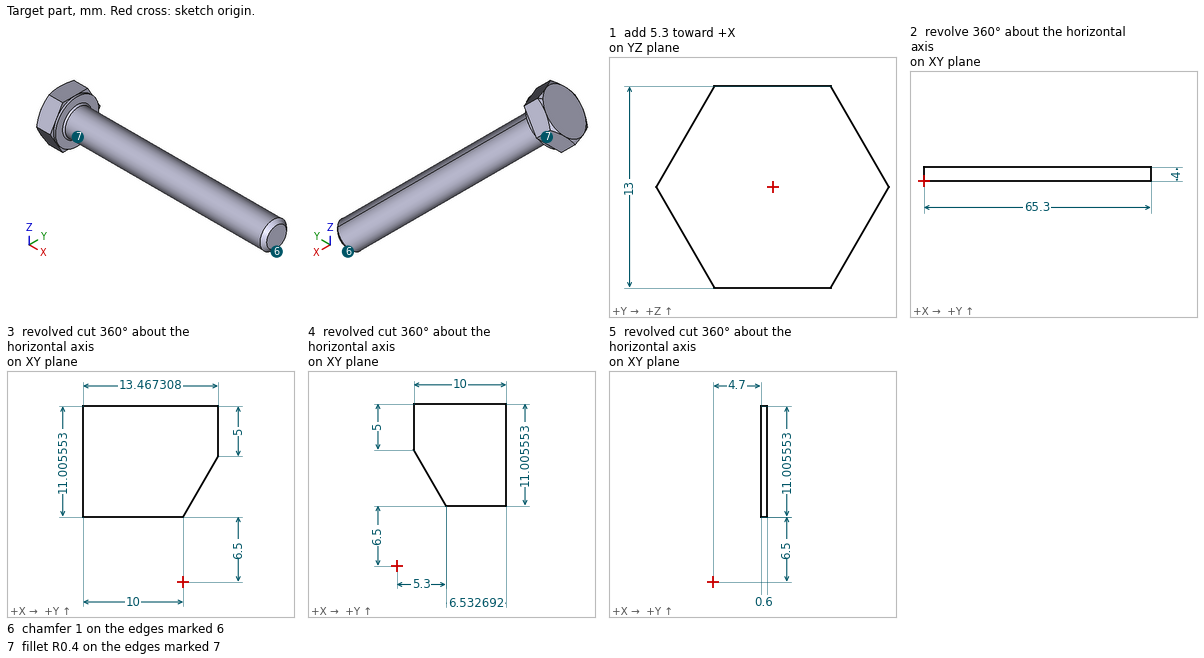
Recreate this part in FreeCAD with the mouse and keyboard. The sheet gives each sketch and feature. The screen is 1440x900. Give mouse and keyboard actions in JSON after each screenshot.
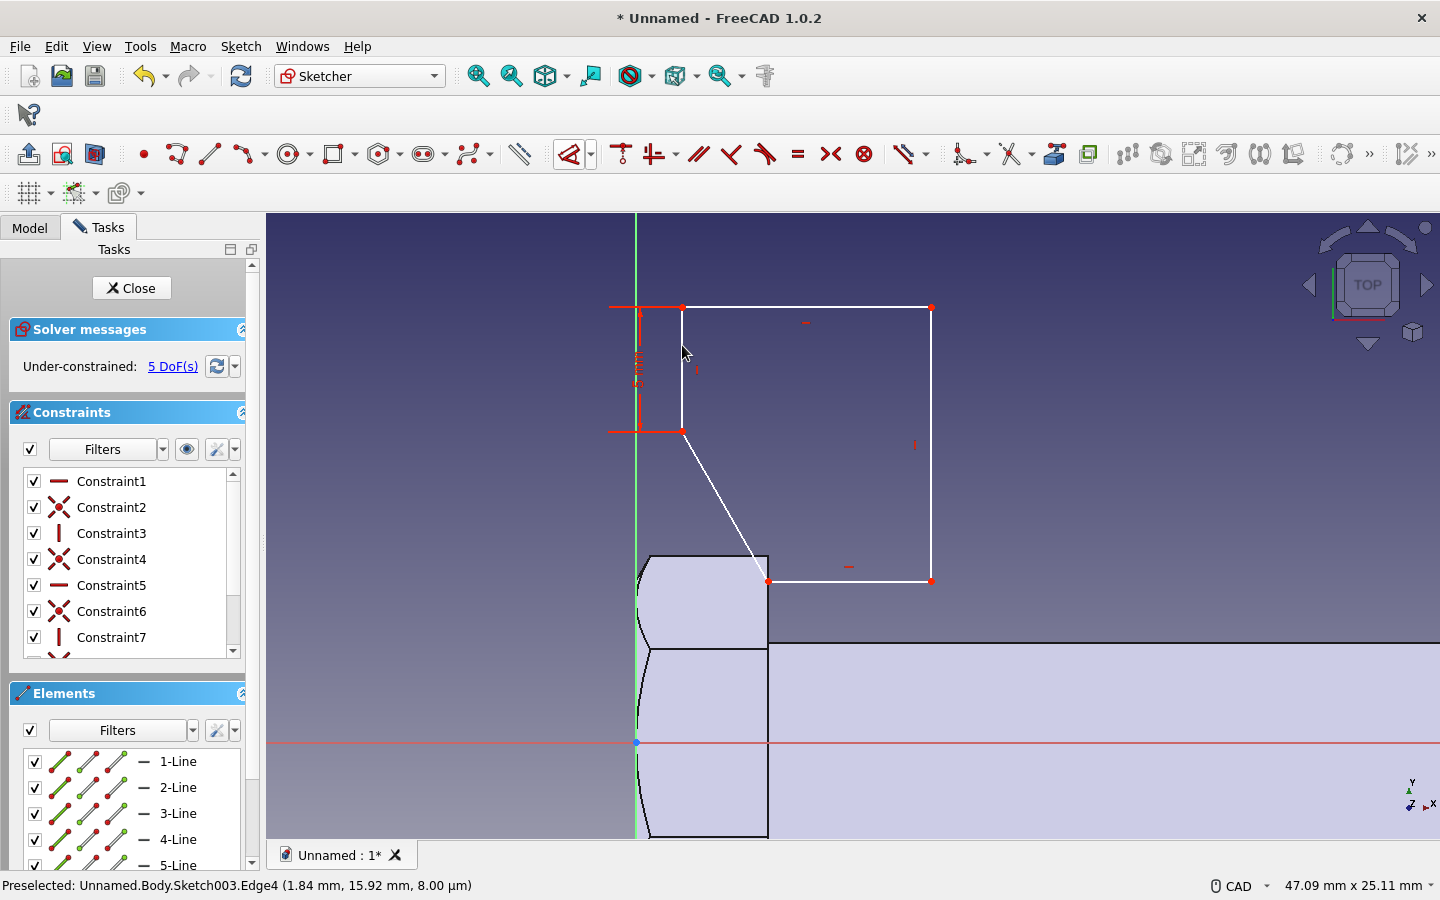
{"action": "left_click", "coordinate": [856, 307]}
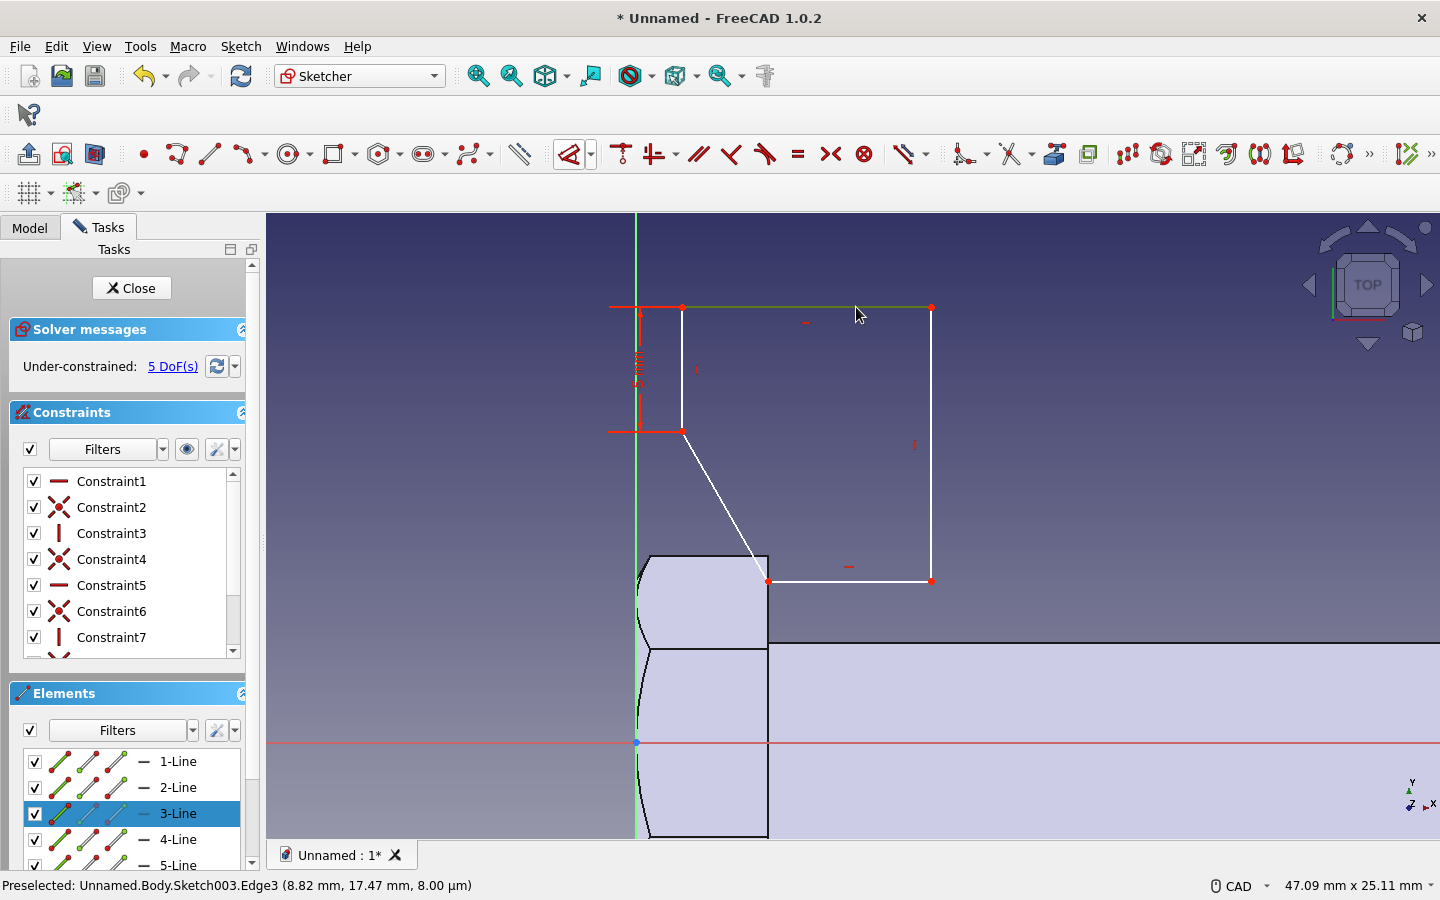
{"action": "left_click", "coordinate": [590, 154]}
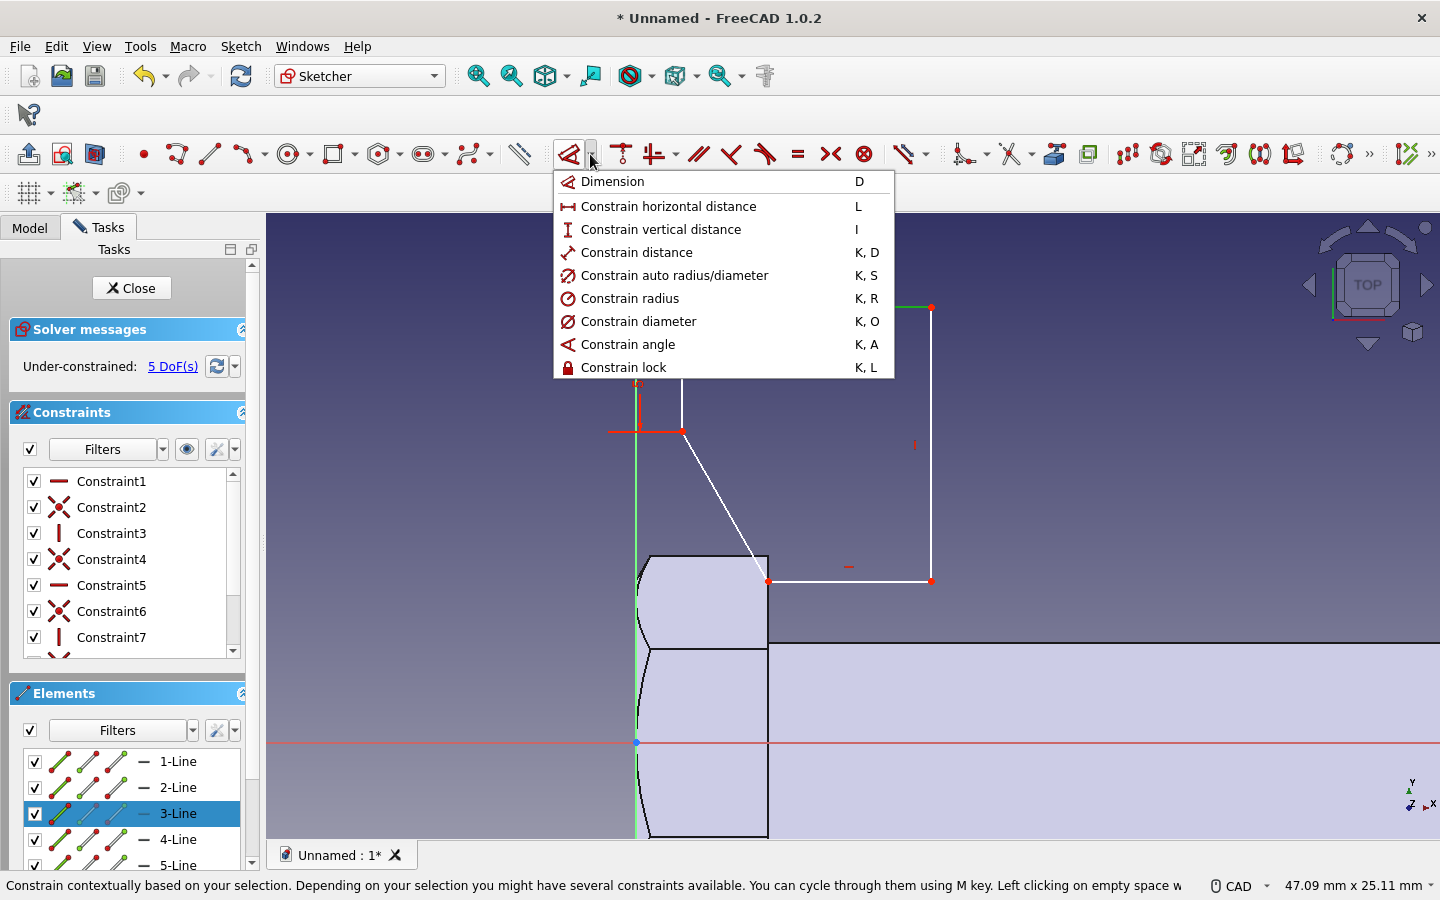
{"action": "left_click", "coordinate": [724, 206]}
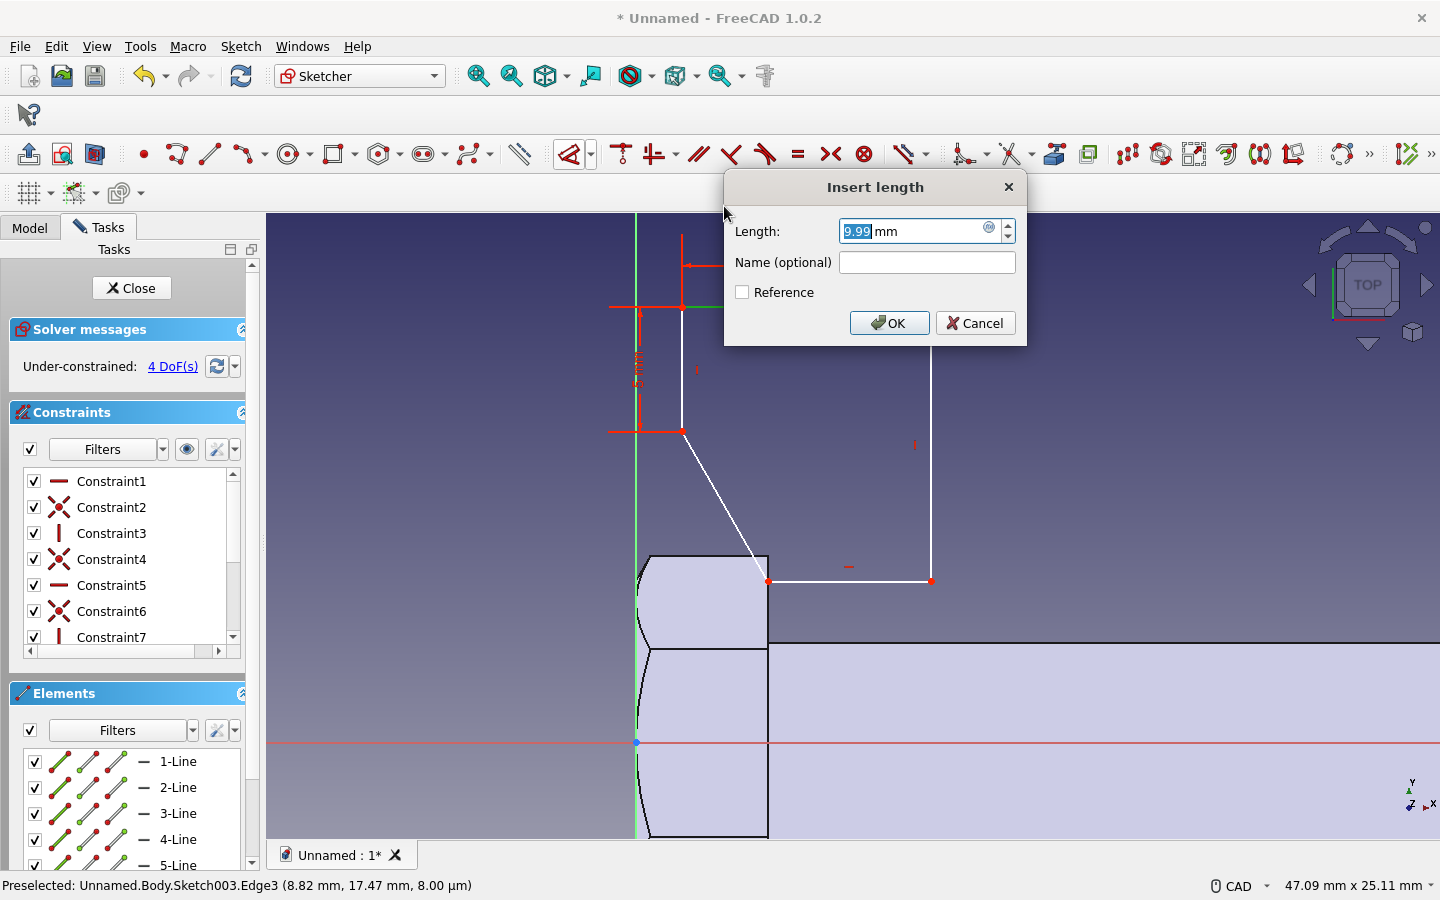
{"action": "type", "text": "10"}
{"action": "key", "text": "Return"}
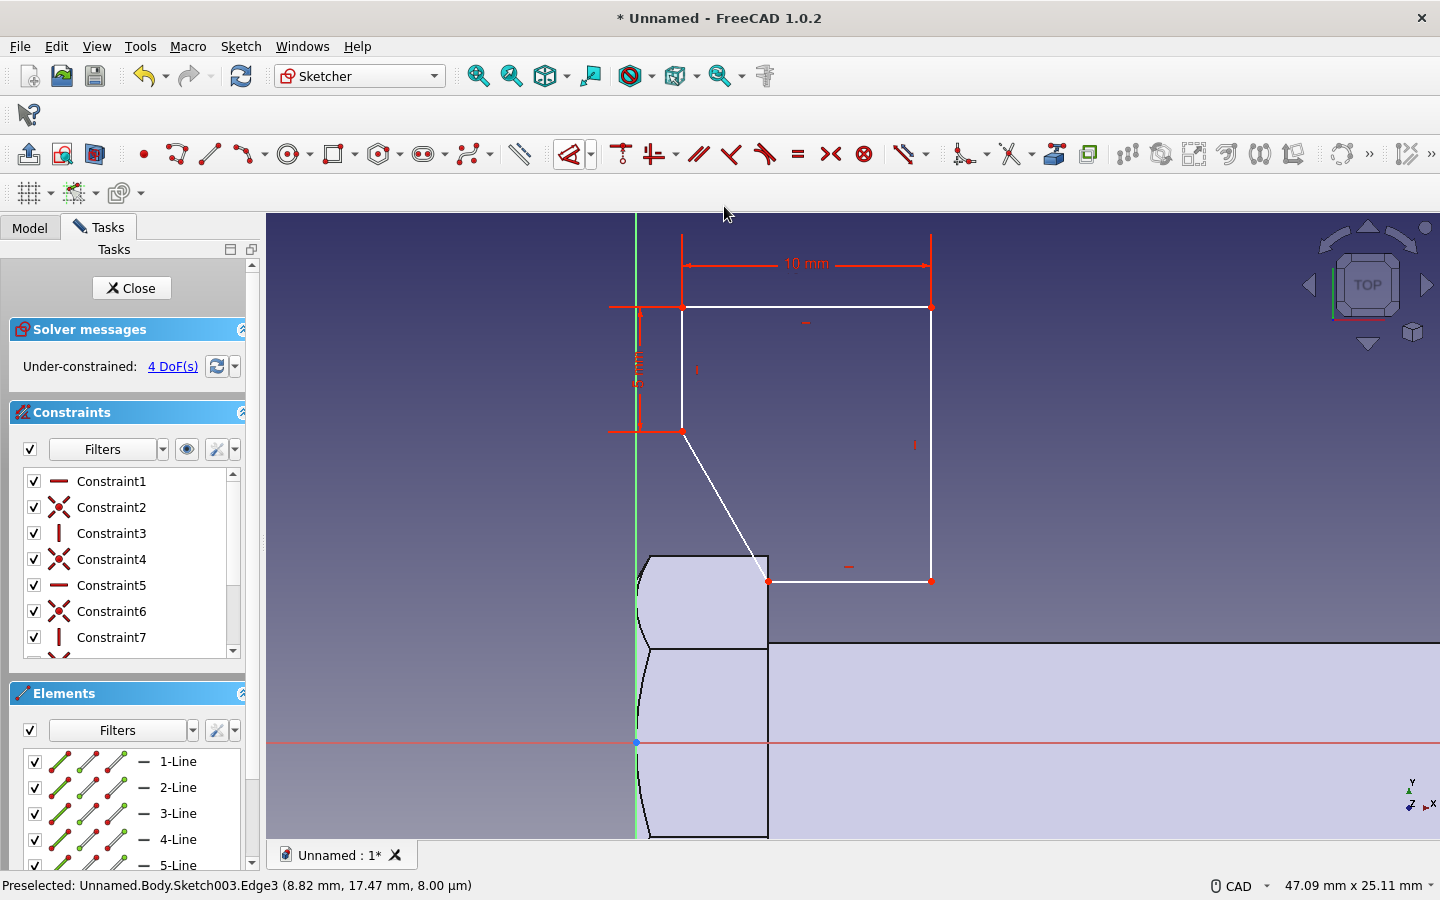
{"action": "left_click", "coordinate": [768, 582]}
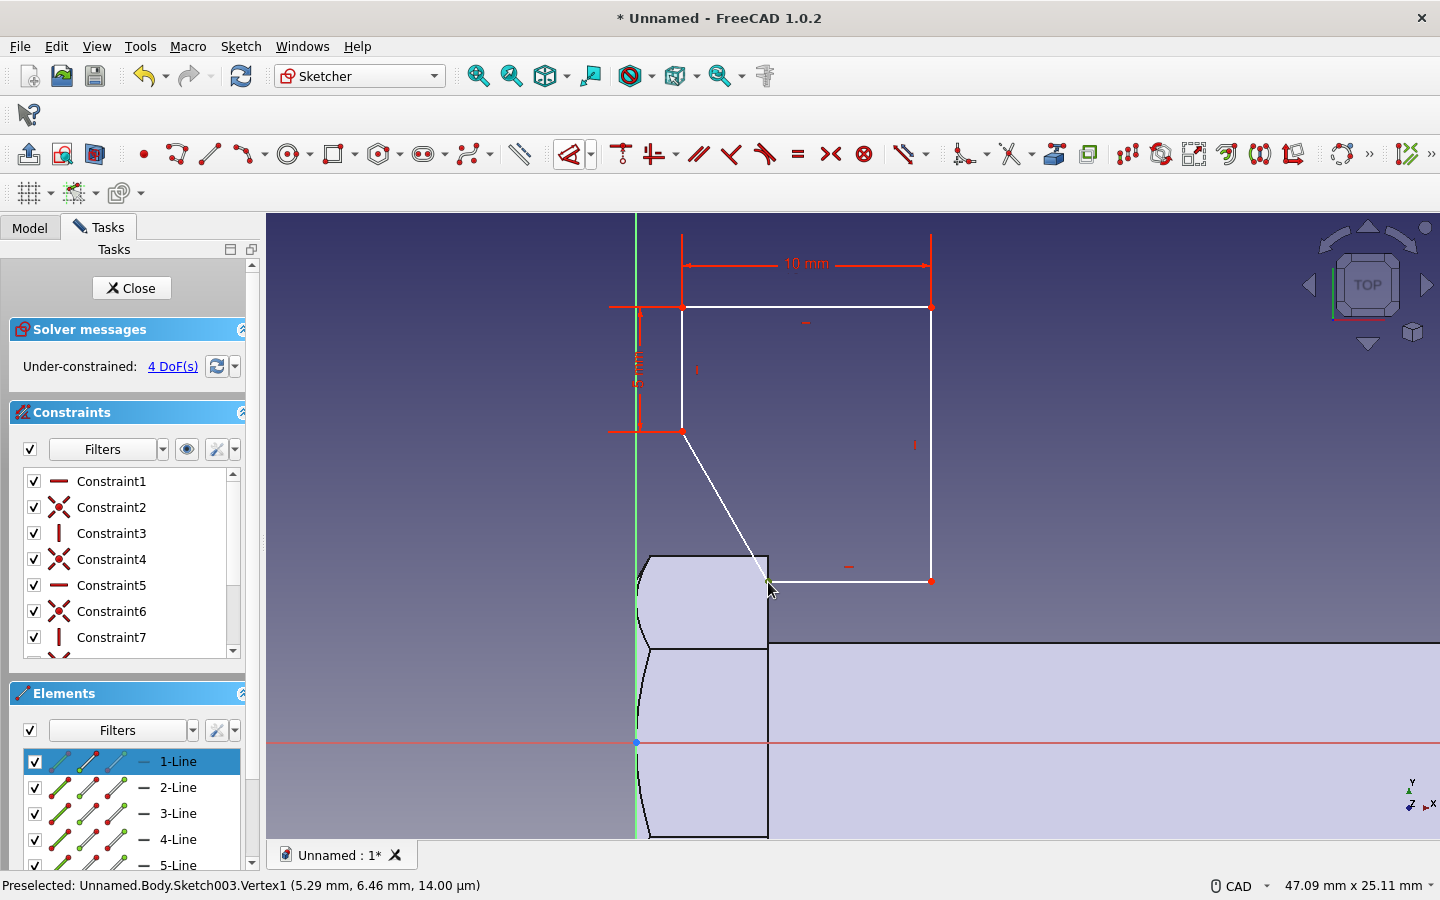
{"action": "left_click", "coordinate": [590, 154]}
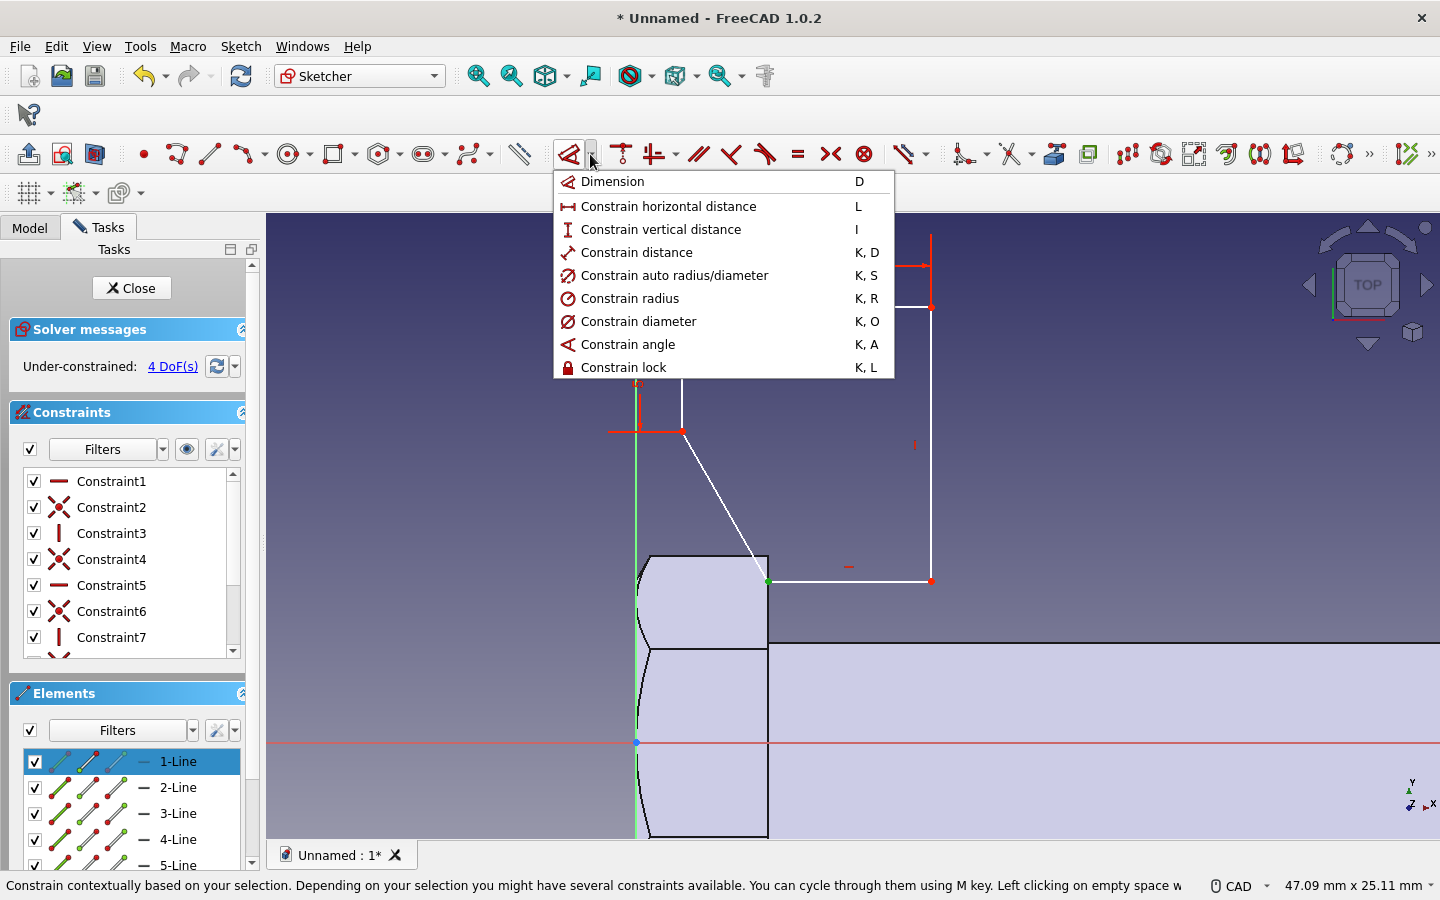
{"action": "left_click", "coordinate": [724, 206]}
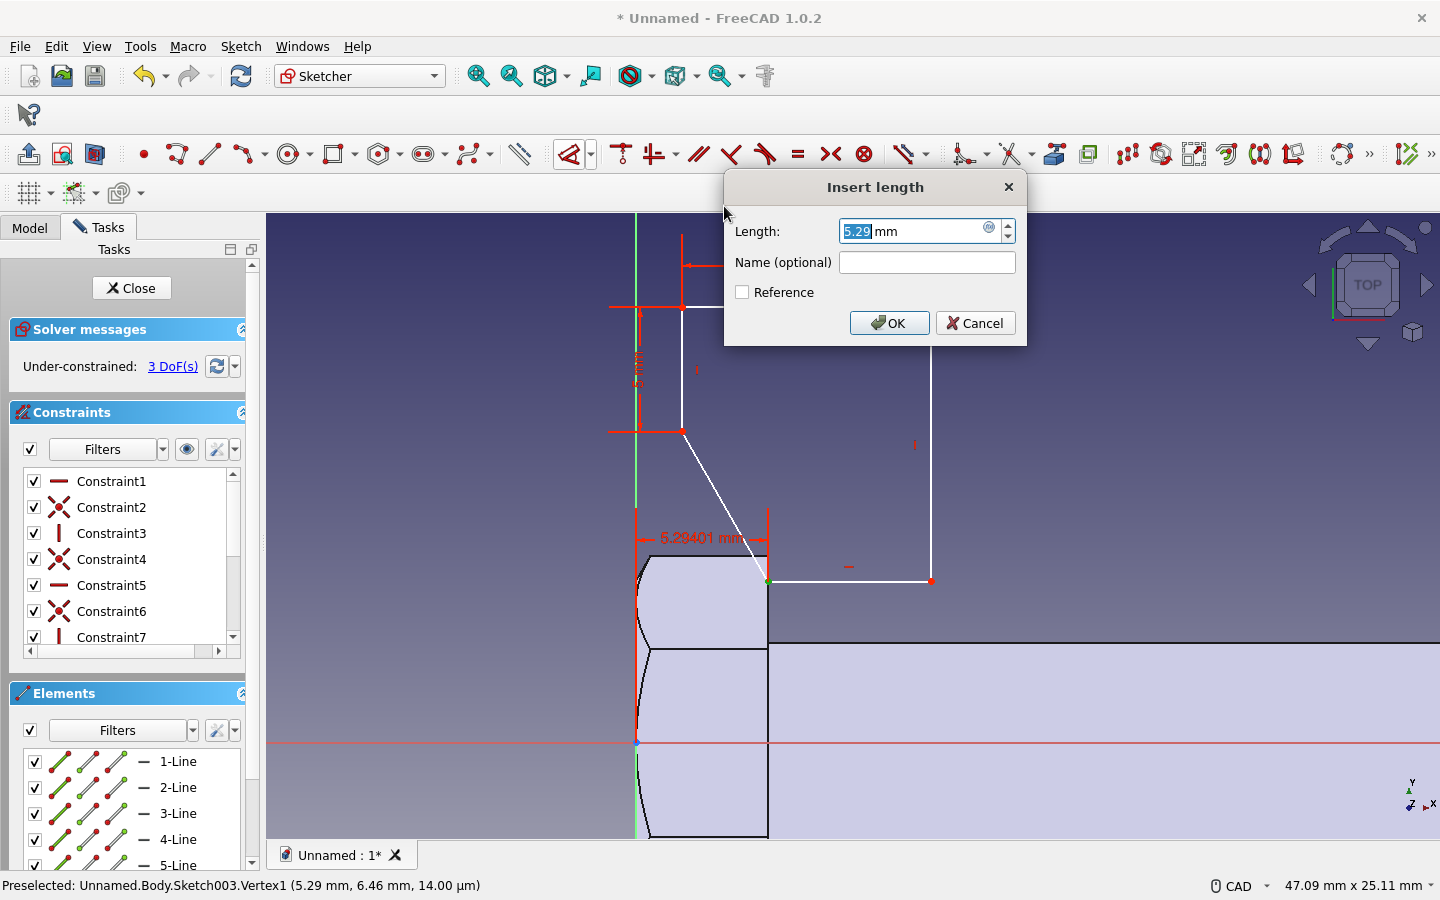
{"action": "type", "text": "5.3"}
{"action": "key", "text": "Return"}